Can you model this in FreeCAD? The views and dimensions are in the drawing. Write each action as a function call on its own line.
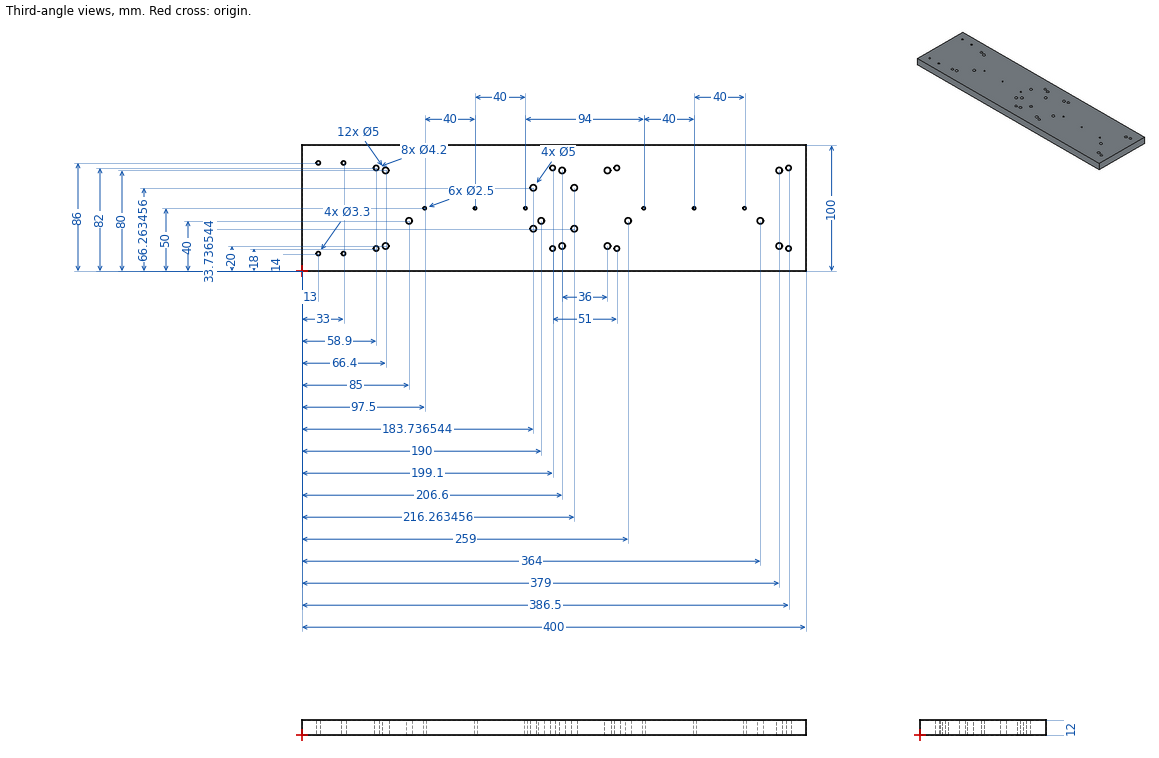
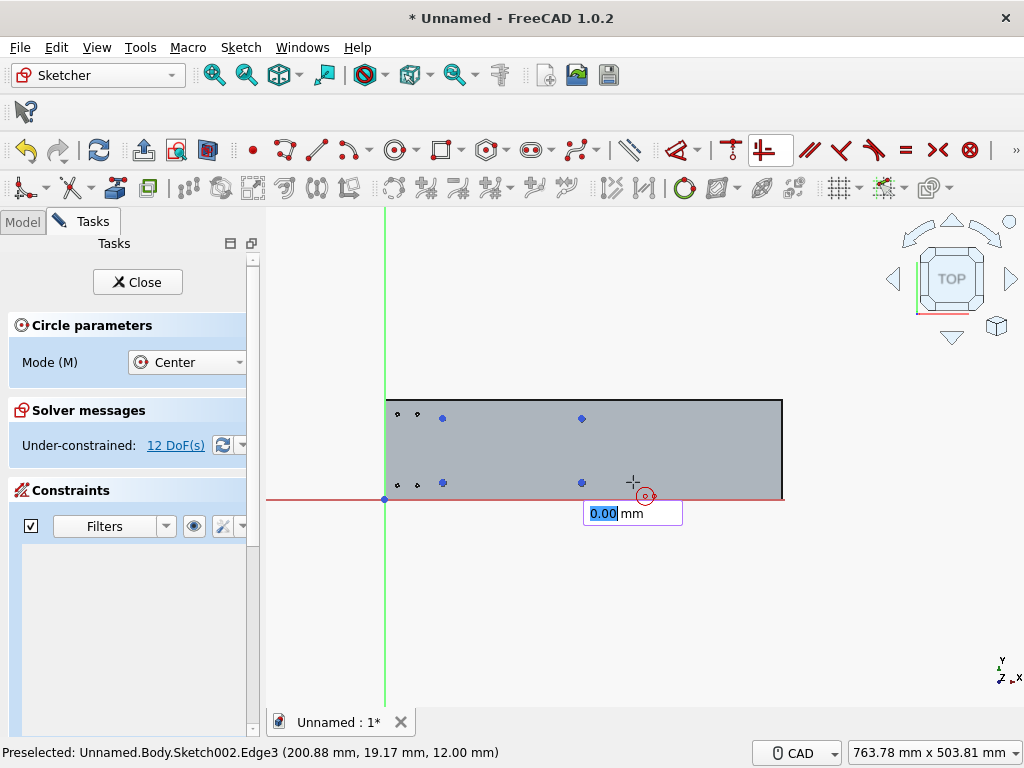
scroll(634, 480, up, 11)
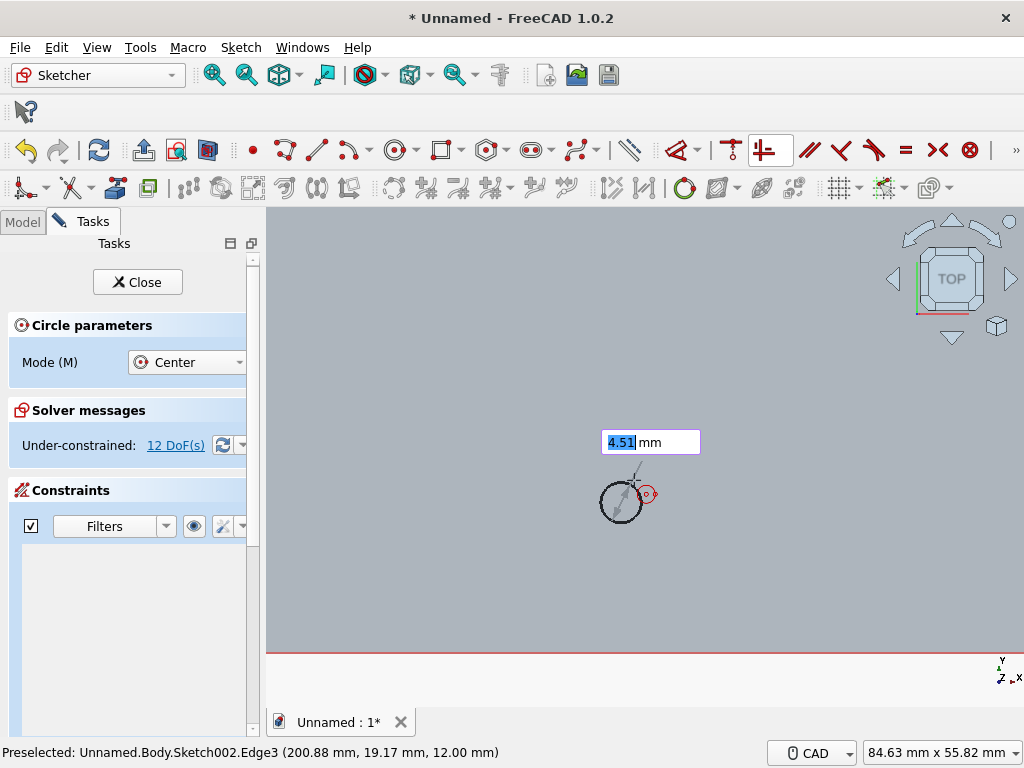
click(632, 478)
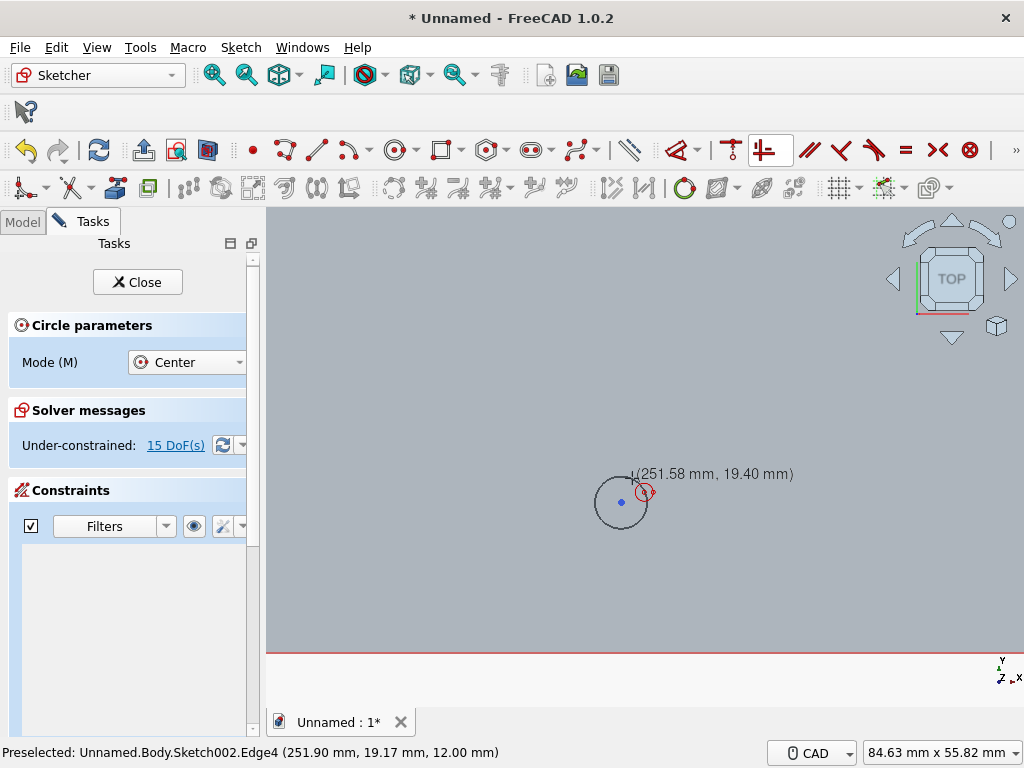
scroll(634, 480, down, 11)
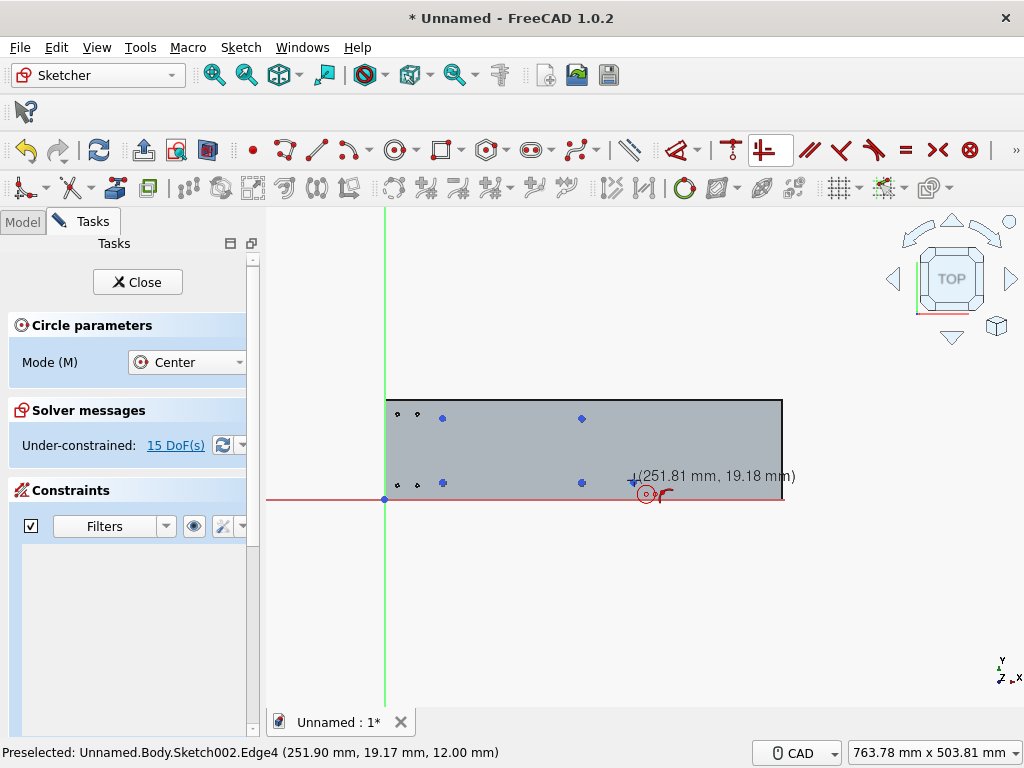
scroll(633, 418, up, 12)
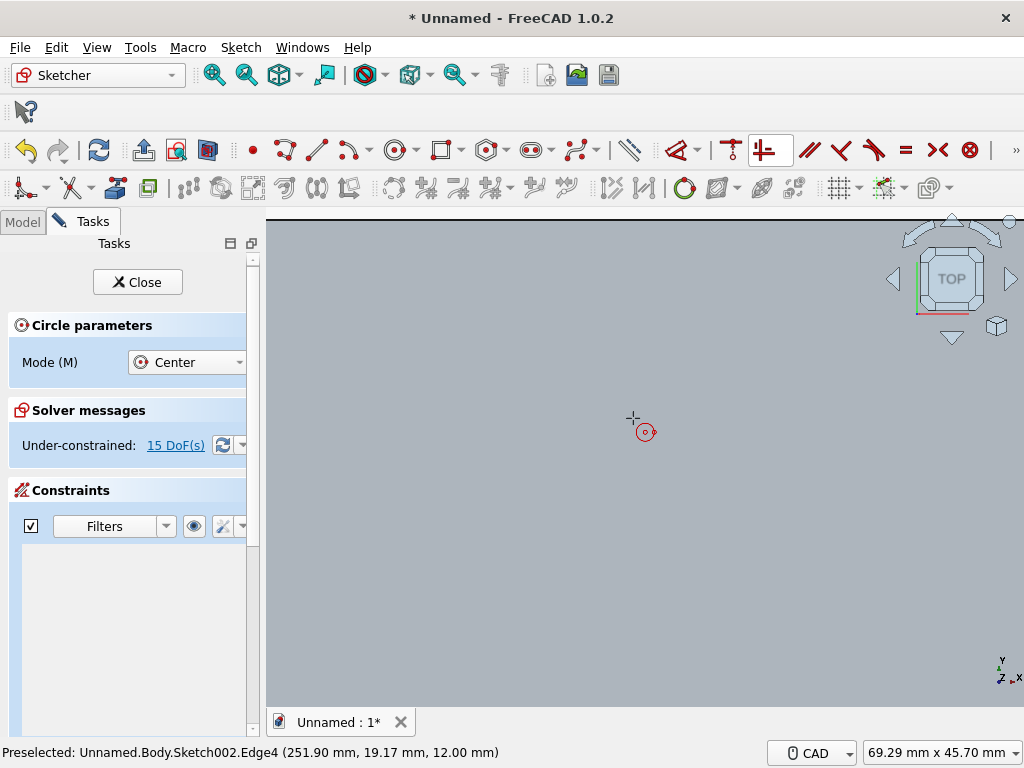
scroll(633, 417, down, 12)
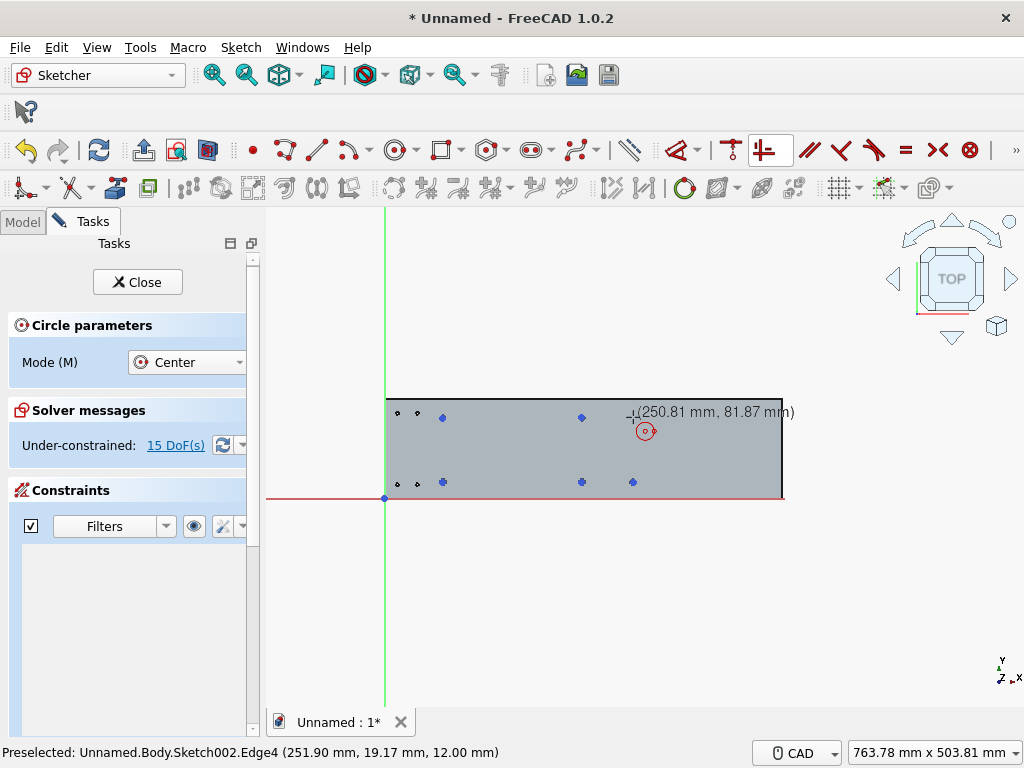
click(633, 417)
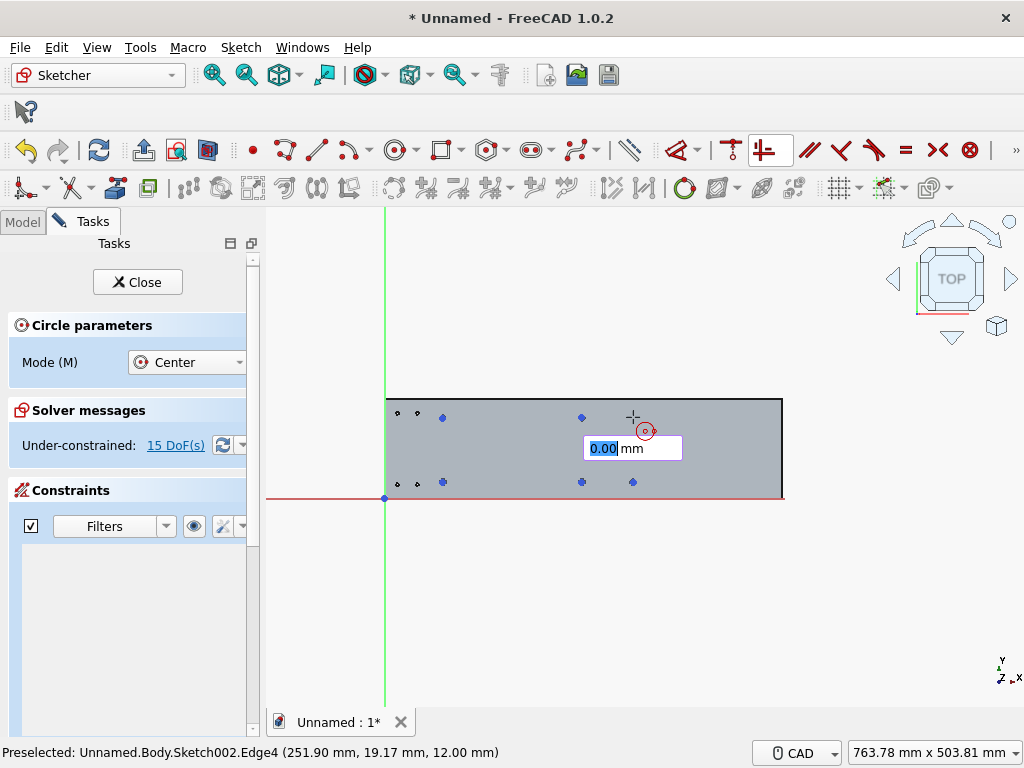
scroll(634, 416, up, 11)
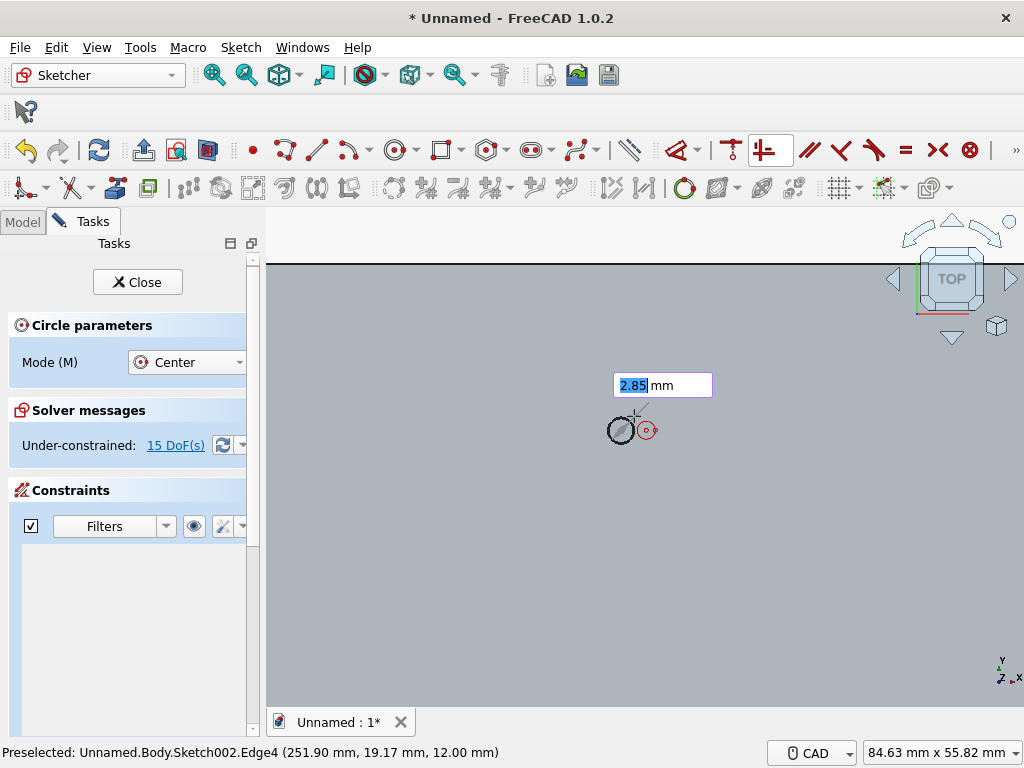
click(632, 411)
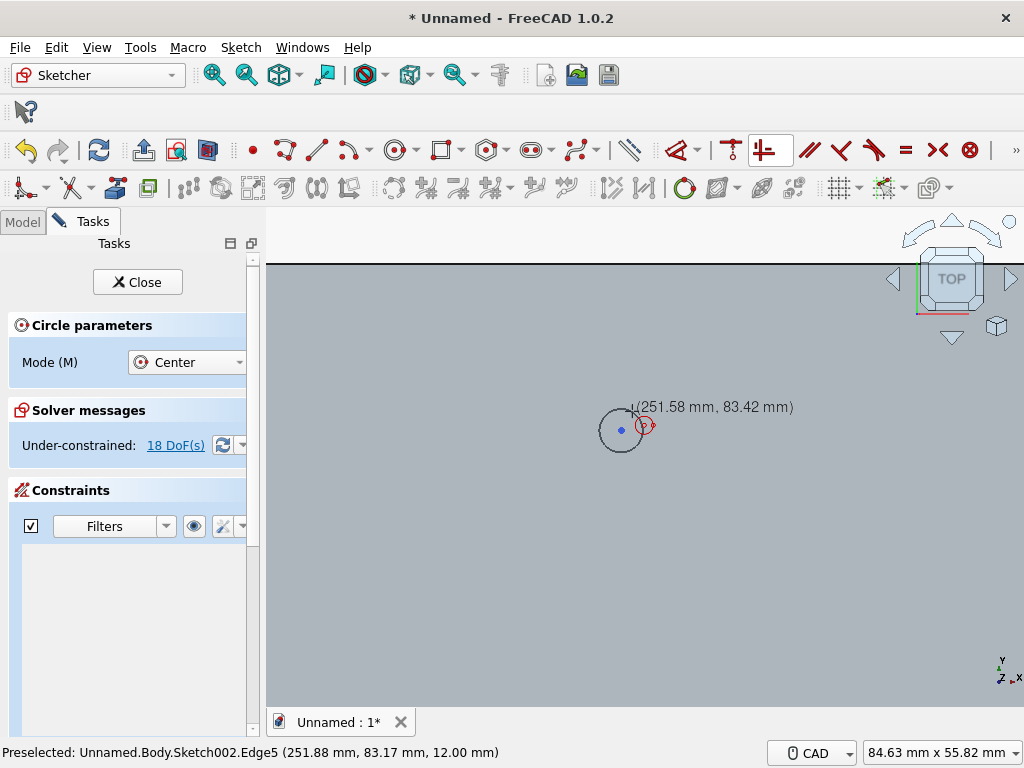
scroll(634, 416, down, 11)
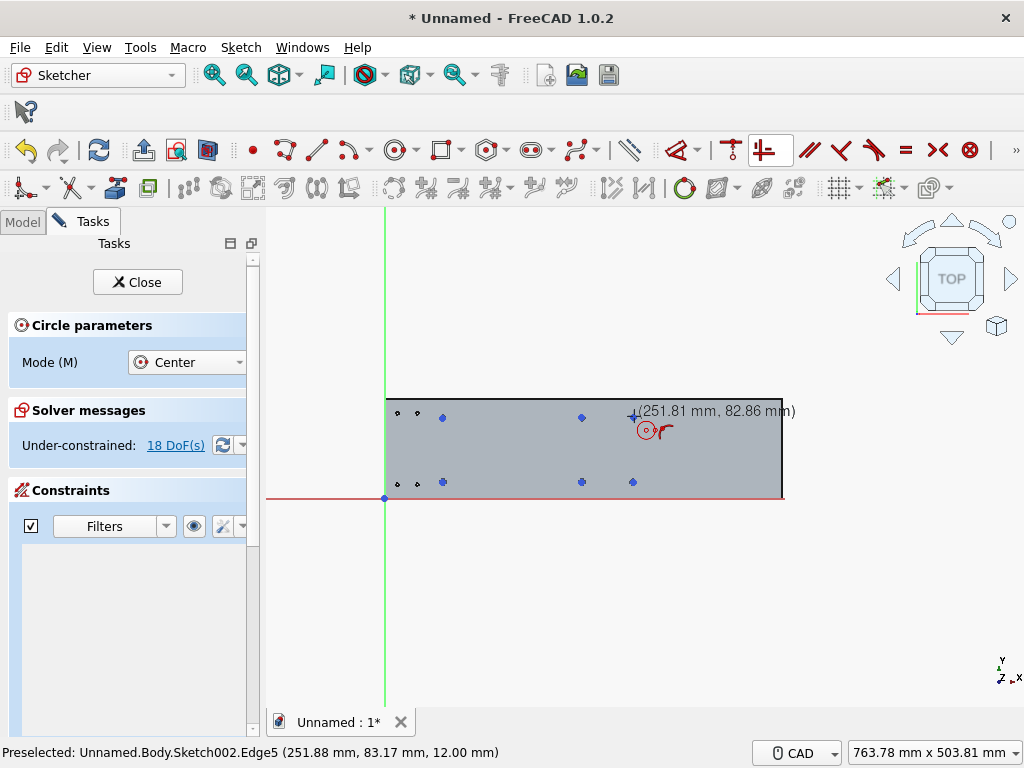
scroll(768, 417, up, 12)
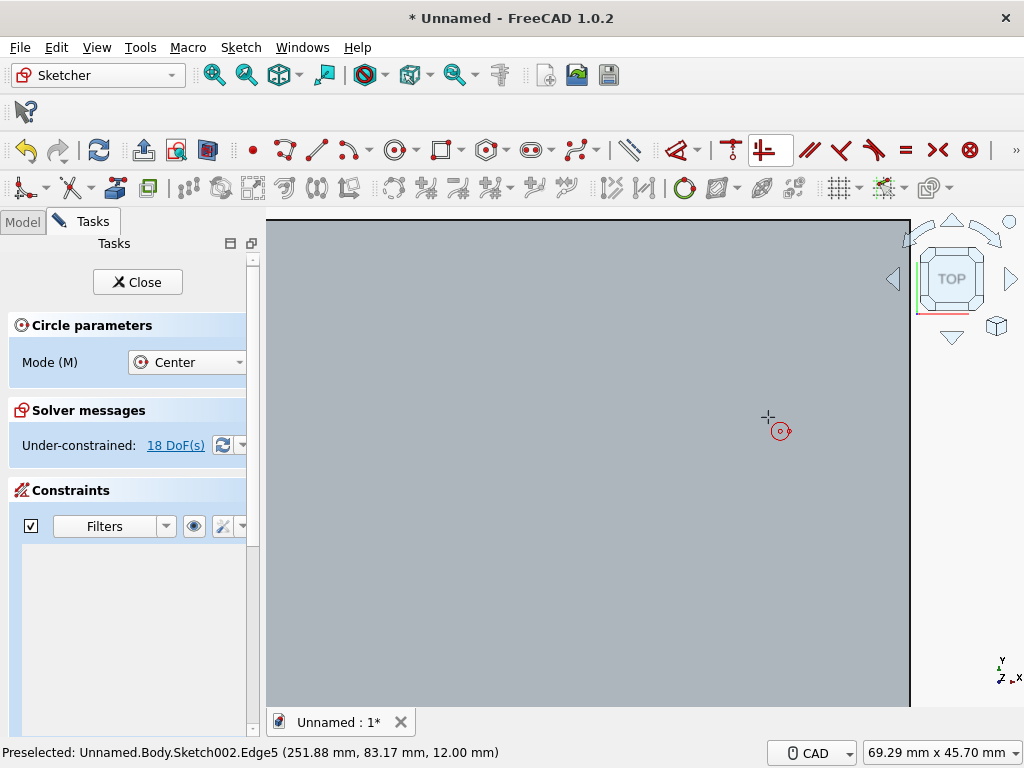
scroll(768, 417, down, 12)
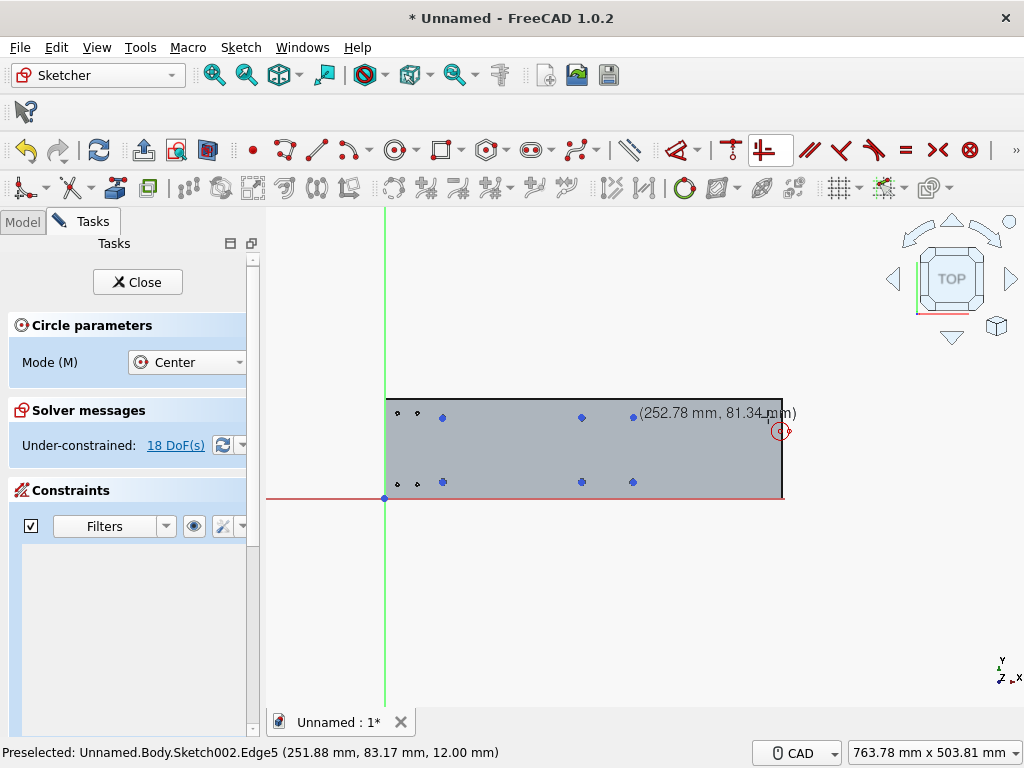
click(768, 417)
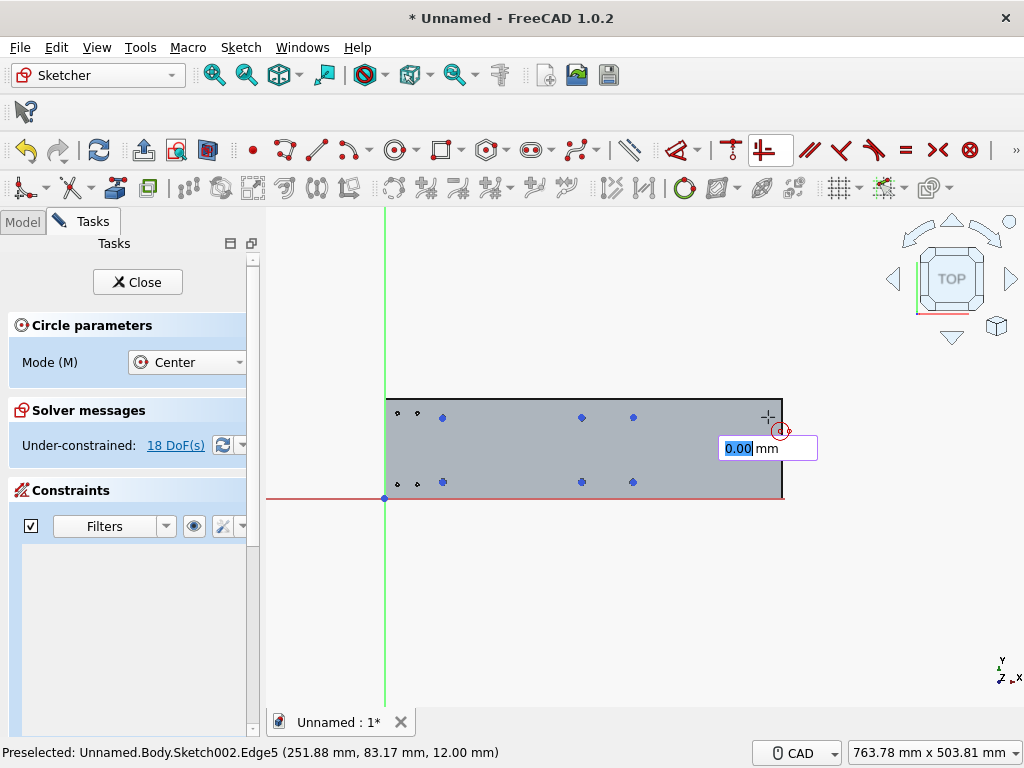
scroll(770, 416, up, 11)